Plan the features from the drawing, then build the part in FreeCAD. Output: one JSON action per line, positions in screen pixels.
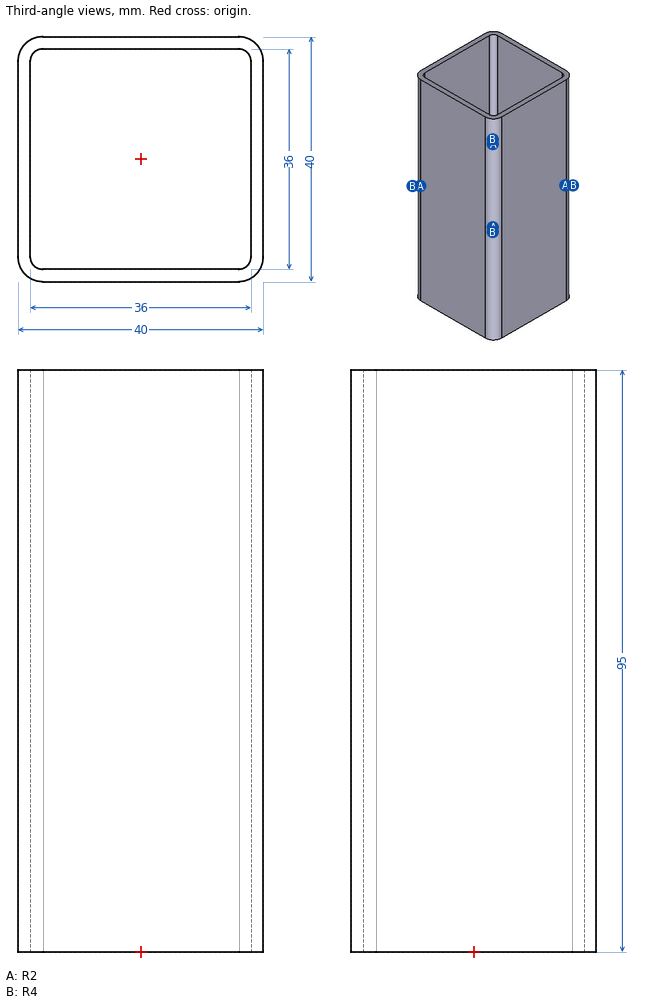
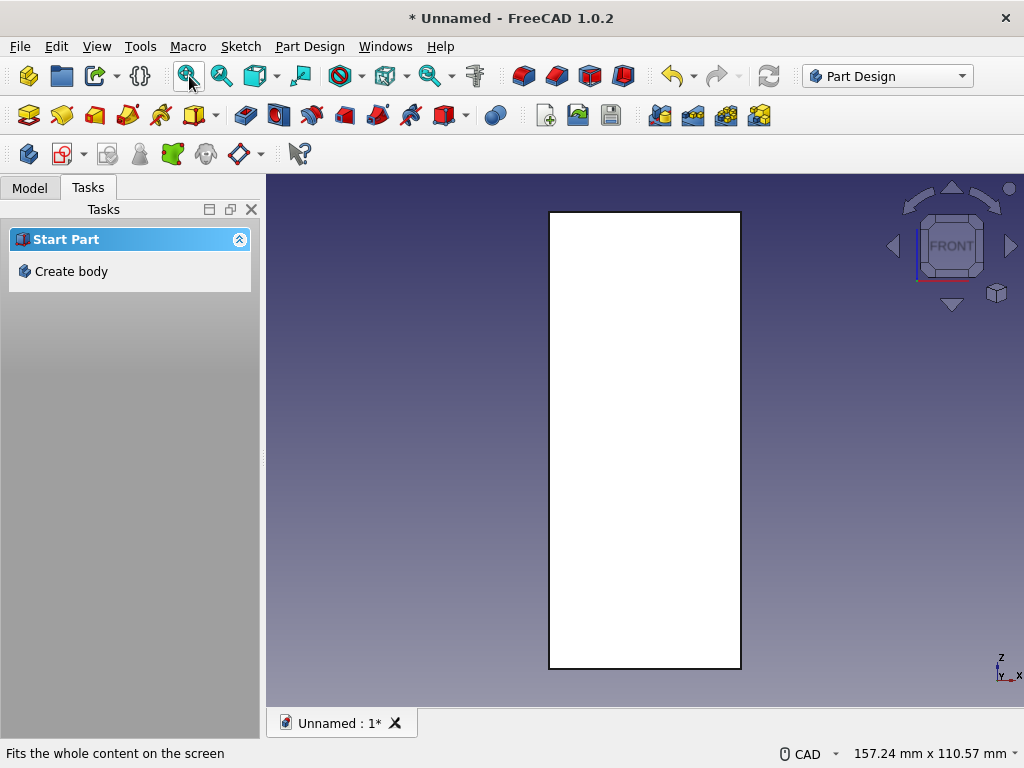
{"action": "key", "text": "3"}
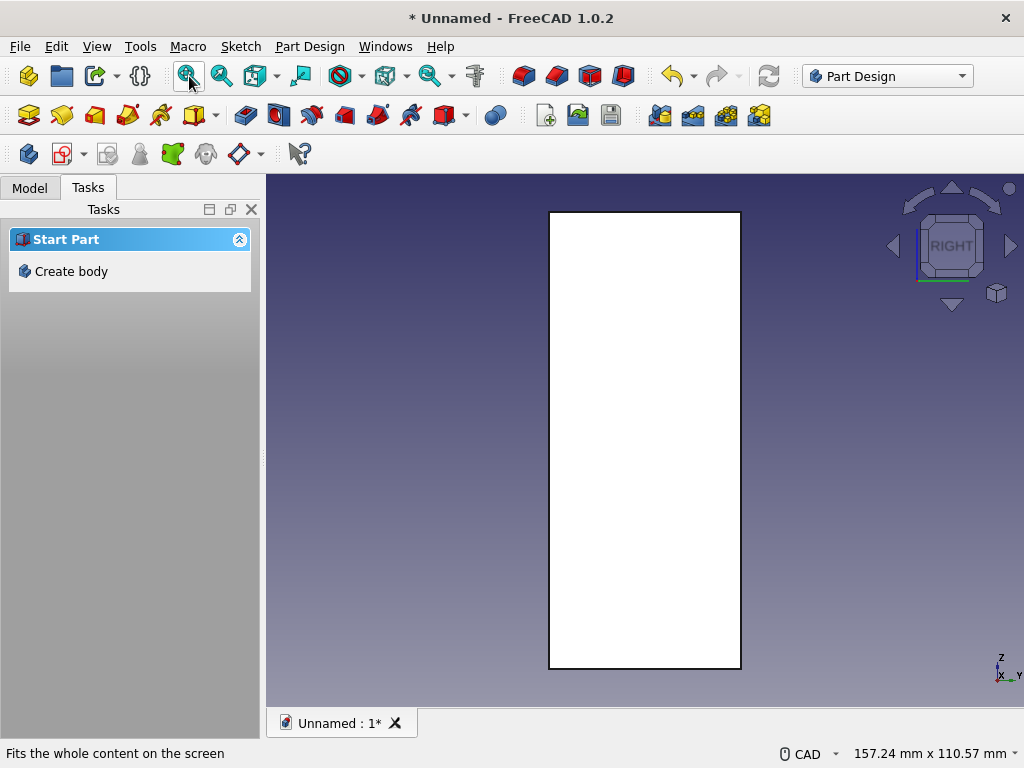
{"action": "key", "text": "5"}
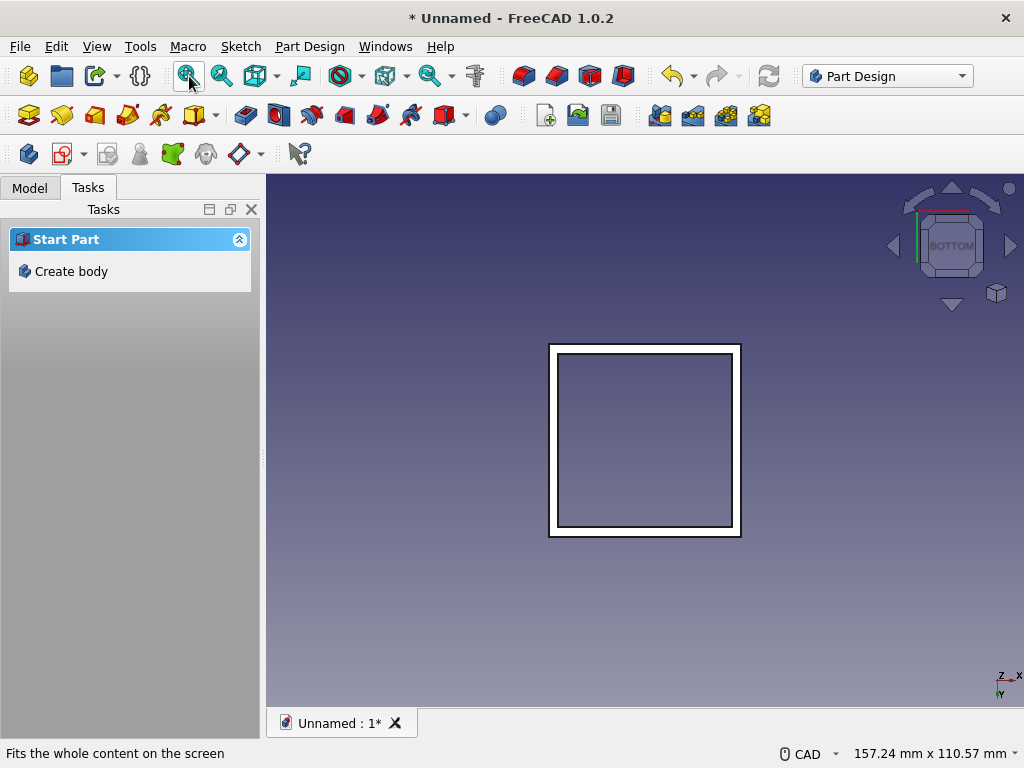
{"action": "left_click", "coordinate": [189, 76]}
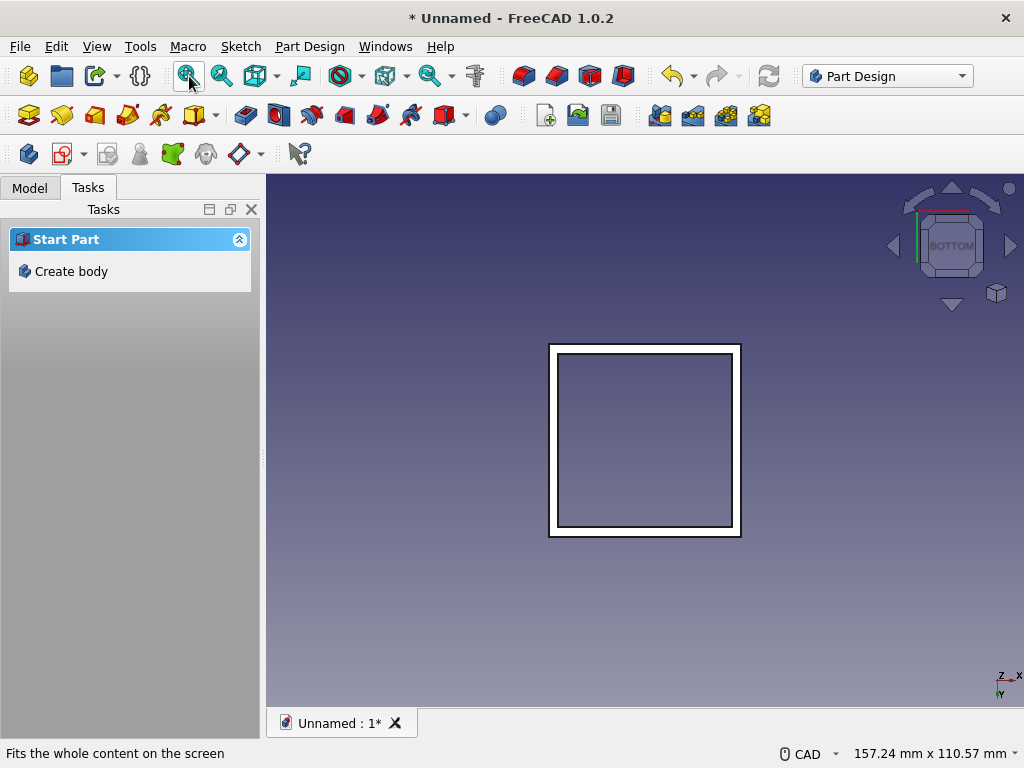
{"action": "key", "text": "4"}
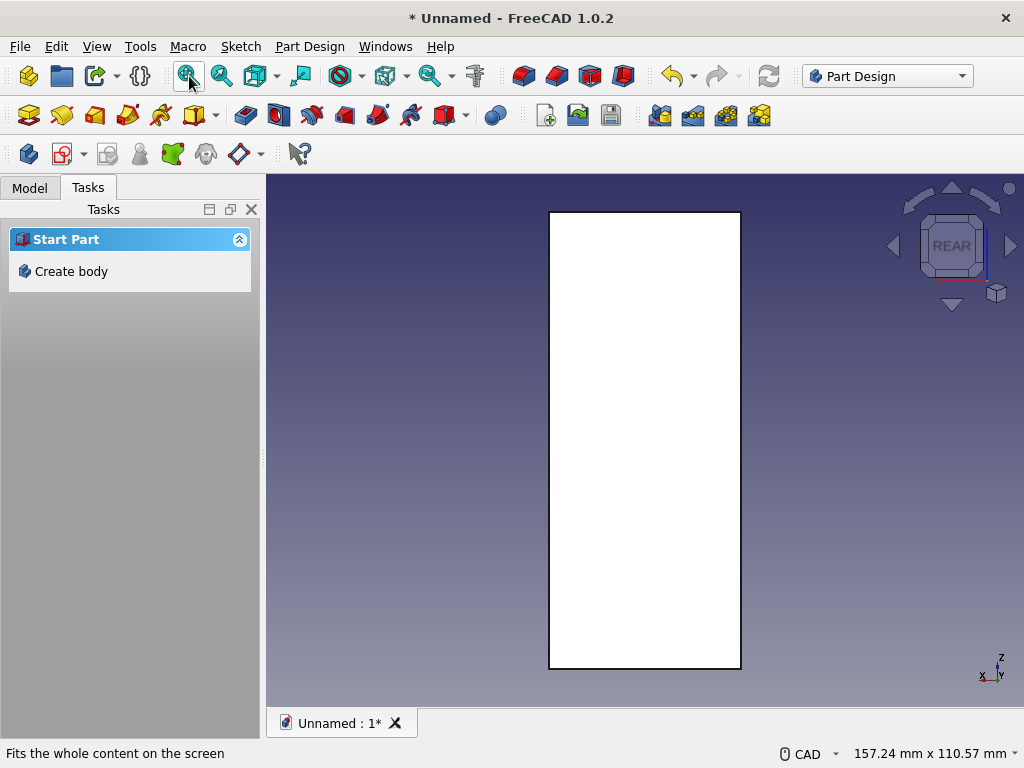
{"action": "key", "text": "6"}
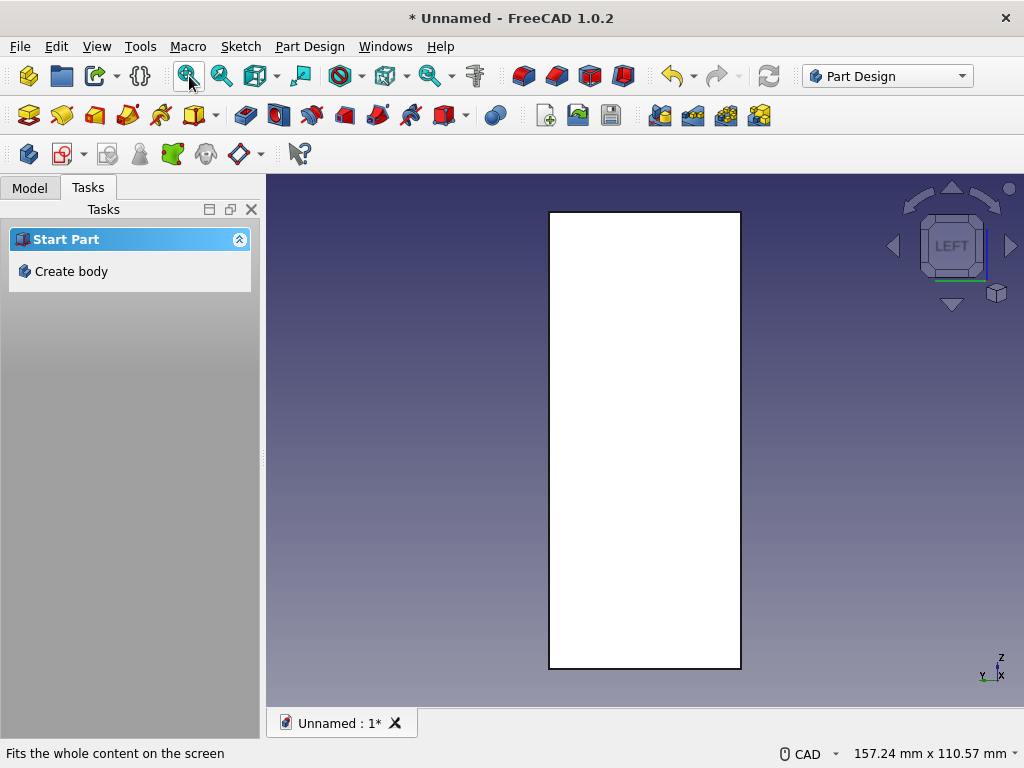
{"action": "key", "text": "v 3"}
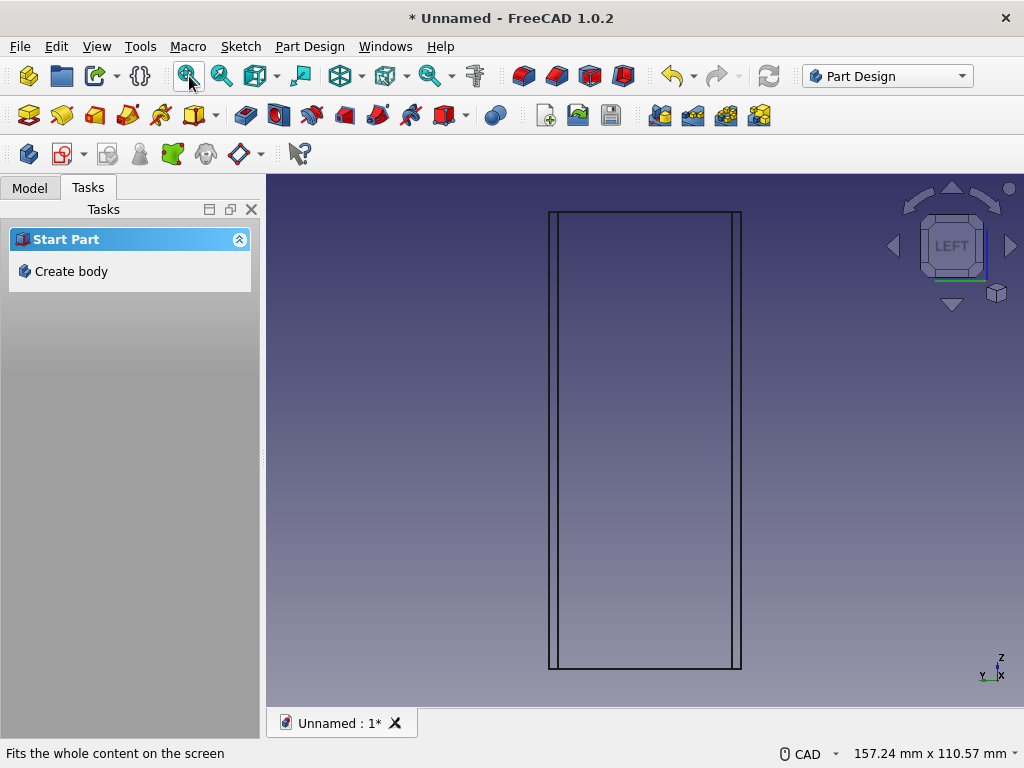
{"action": "key", "text": "0"}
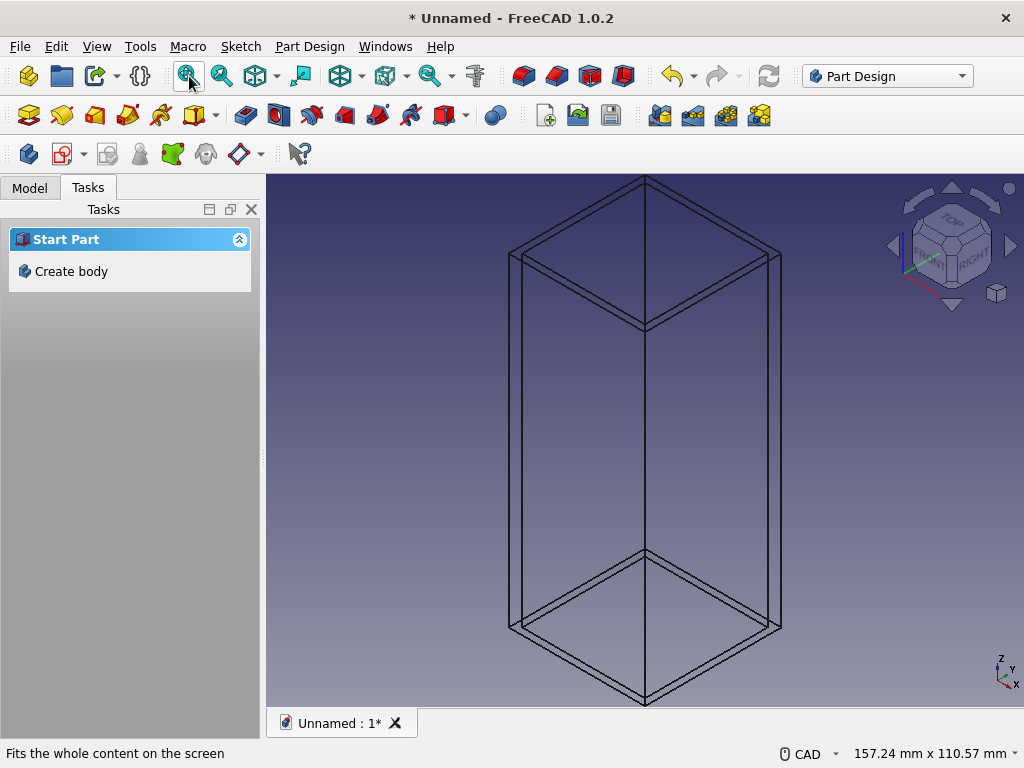
{"action": "left_click", "coordinate": [768, 439]}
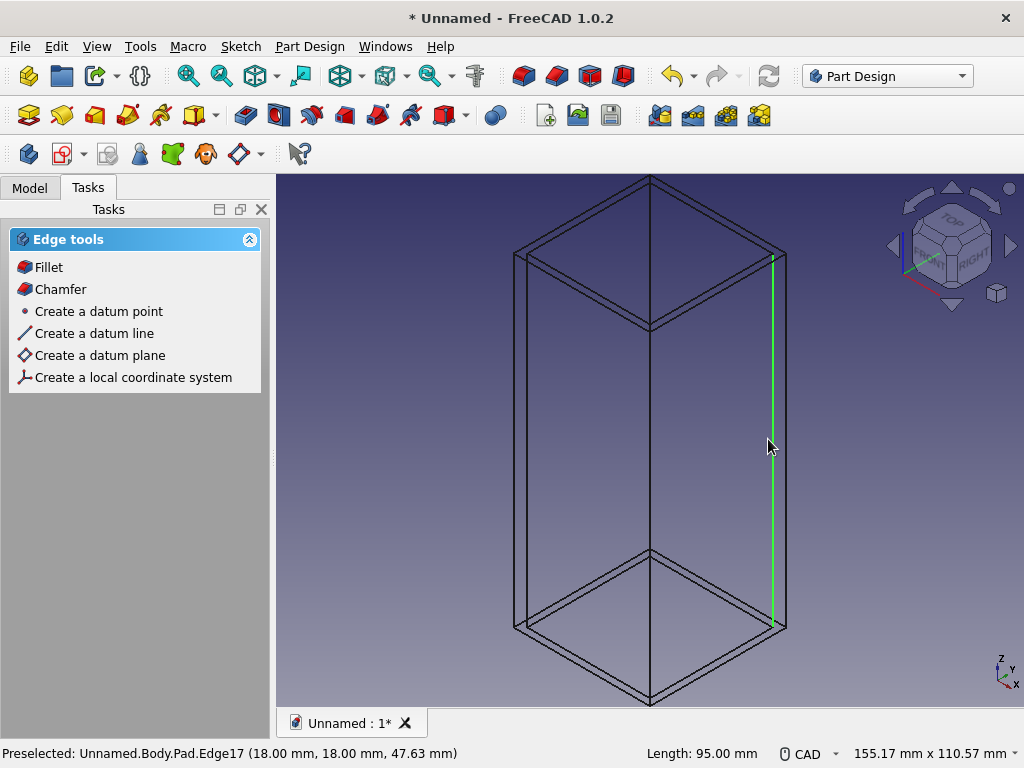
{"action": "left_click", "coordinate": [650, 294], "text": "ctrl"}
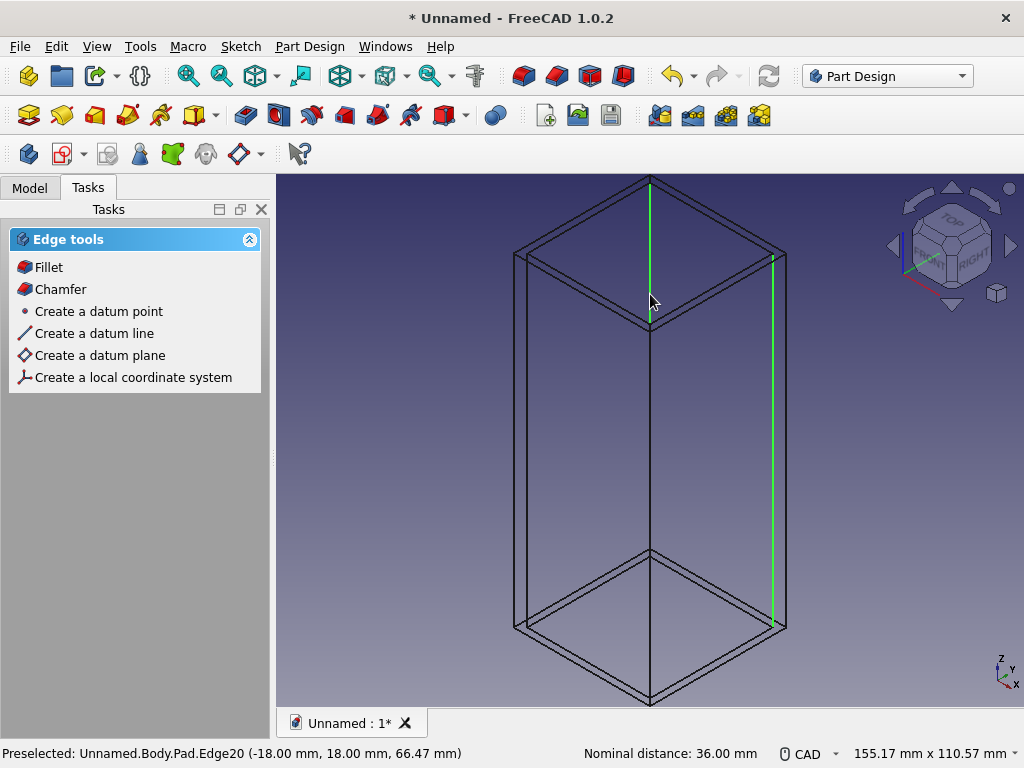
{"action": "left_click", "coordinate": [527, 440], "text": "ctrl"}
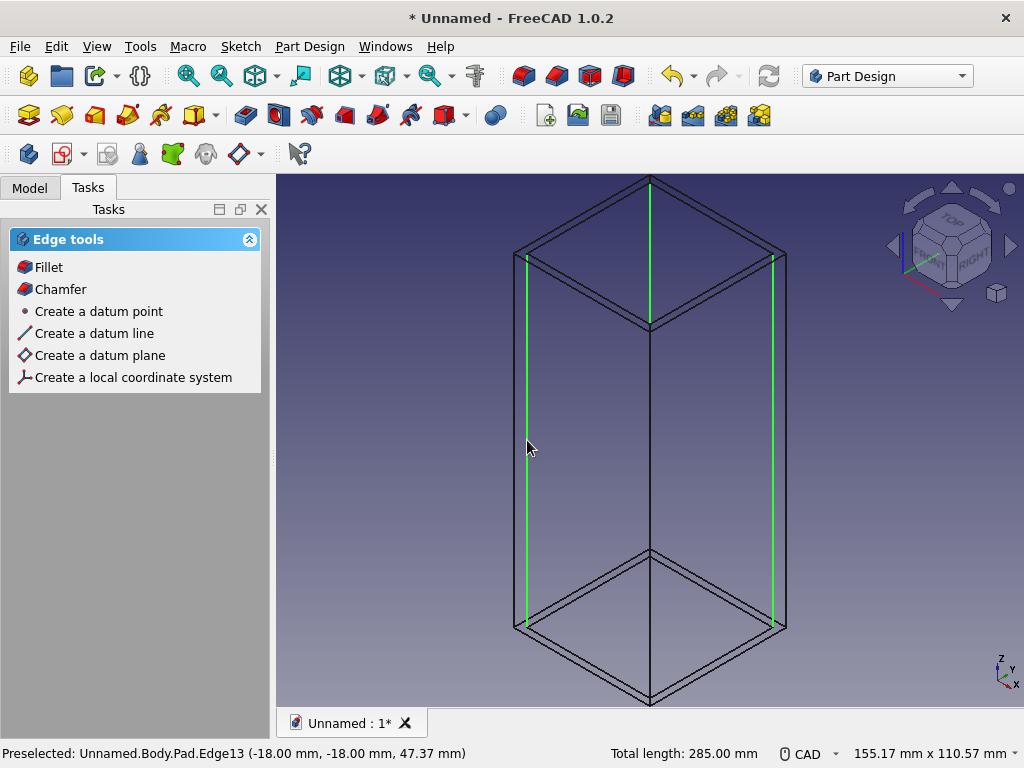
{"action": "scroll", "coordinate": [650, 510], "scroll_direction": "up", "scroll_amount": 6}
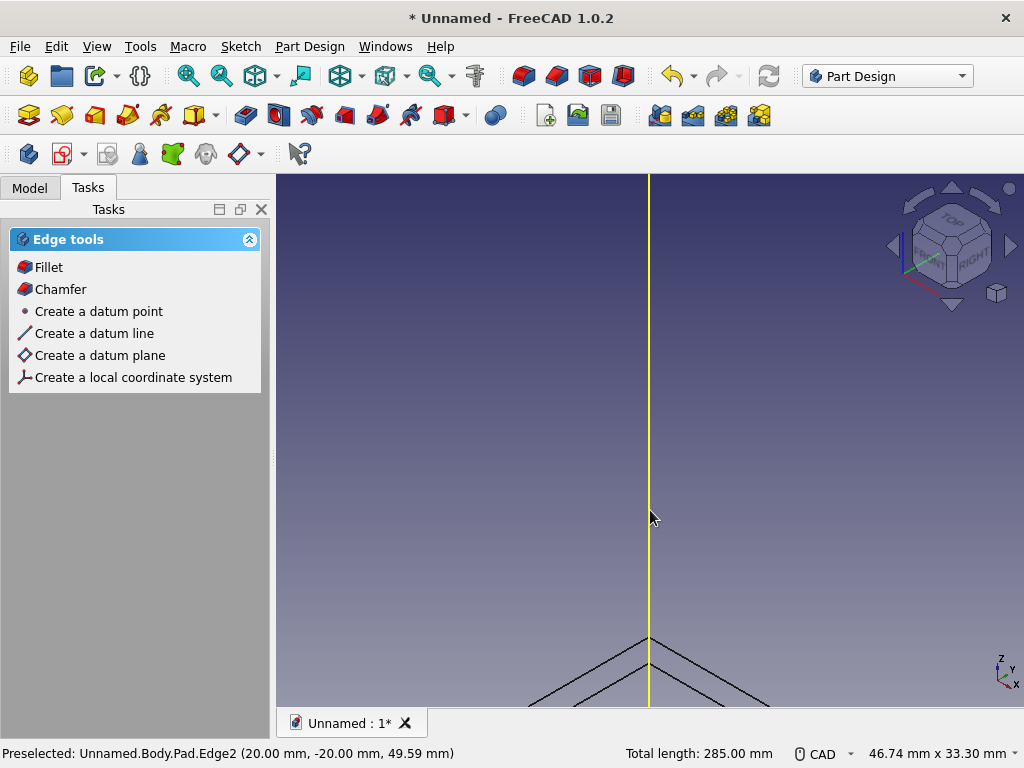
{"action": "left_click", "coordinate": [189, 76]}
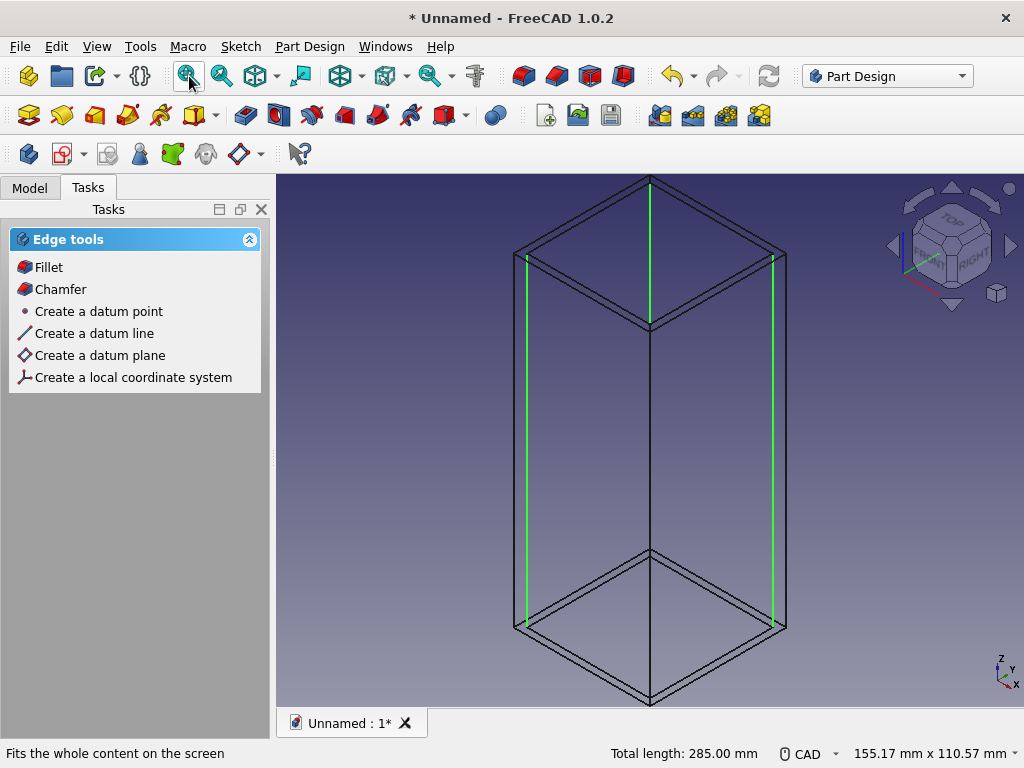
{"action": "key", "text": "2"}